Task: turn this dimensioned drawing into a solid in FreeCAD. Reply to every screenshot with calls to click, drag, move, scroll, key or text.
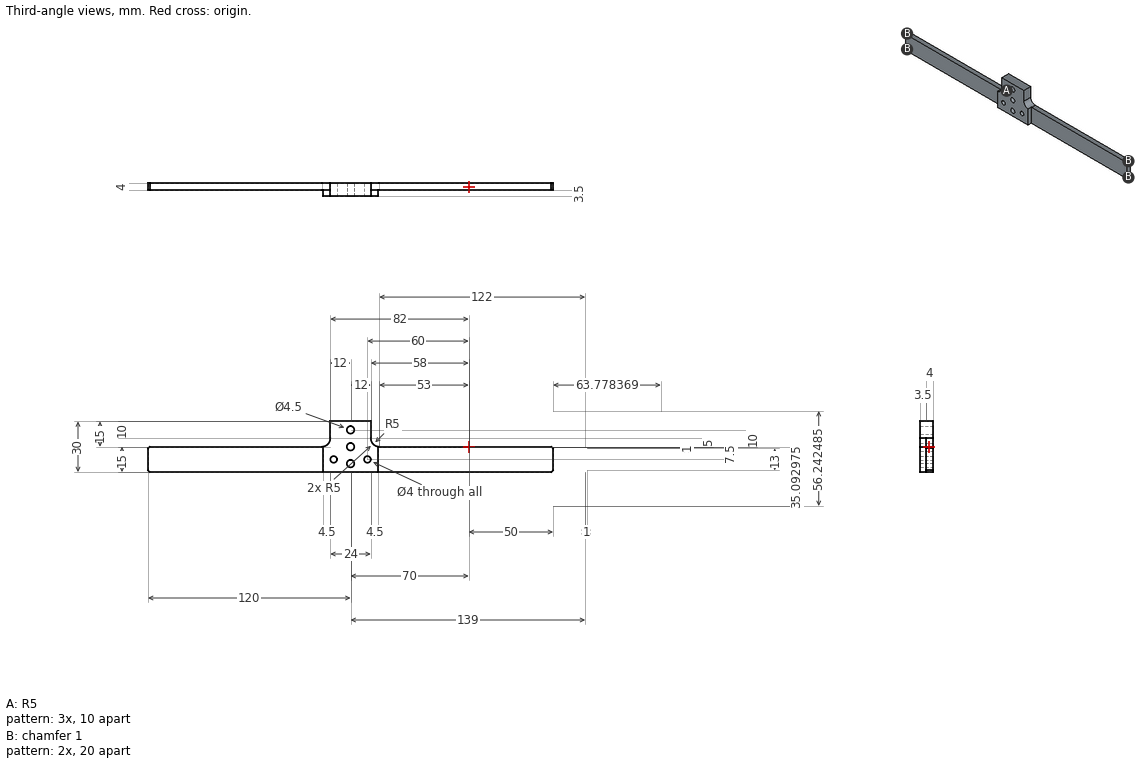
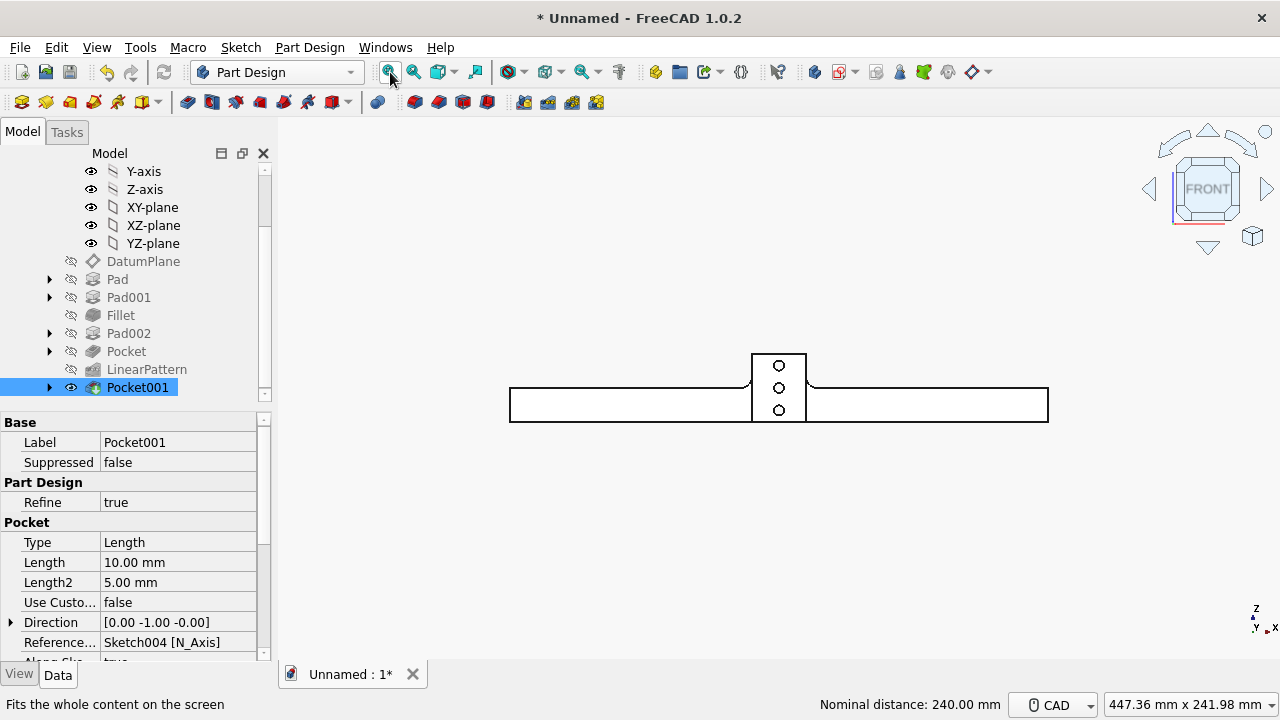
scroll(1048, 421, up, 8)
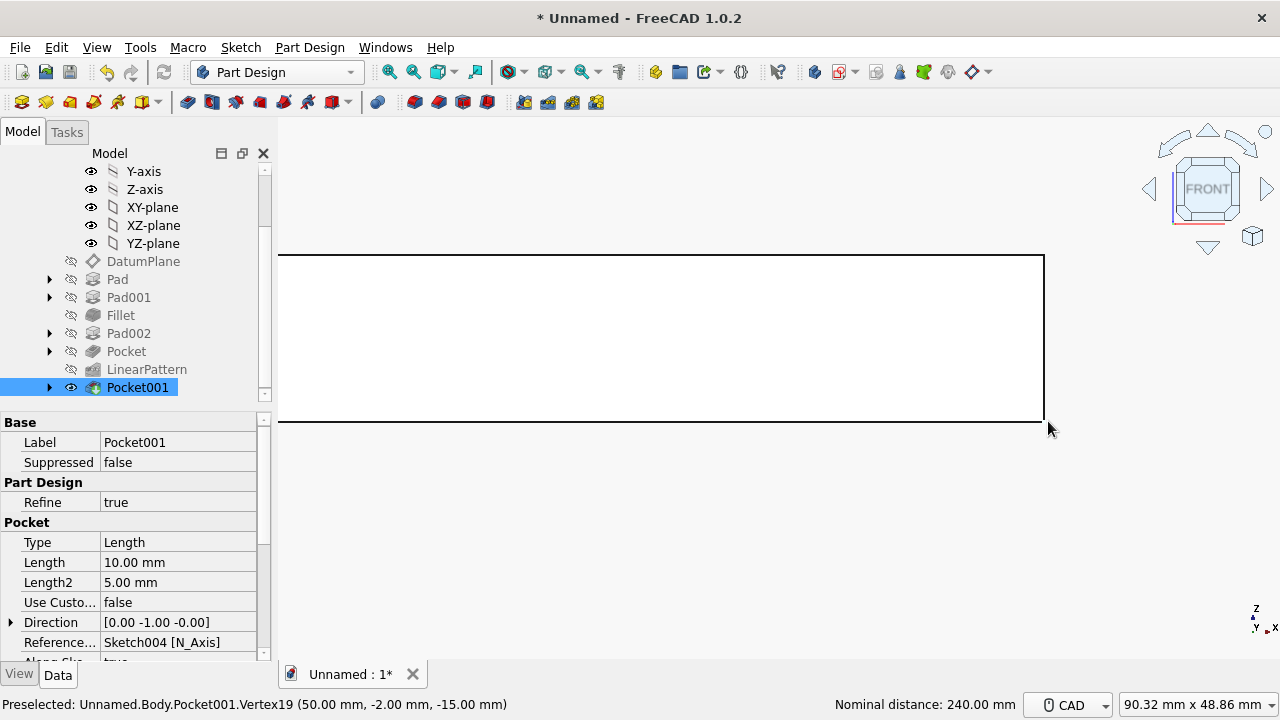
click(390, 72)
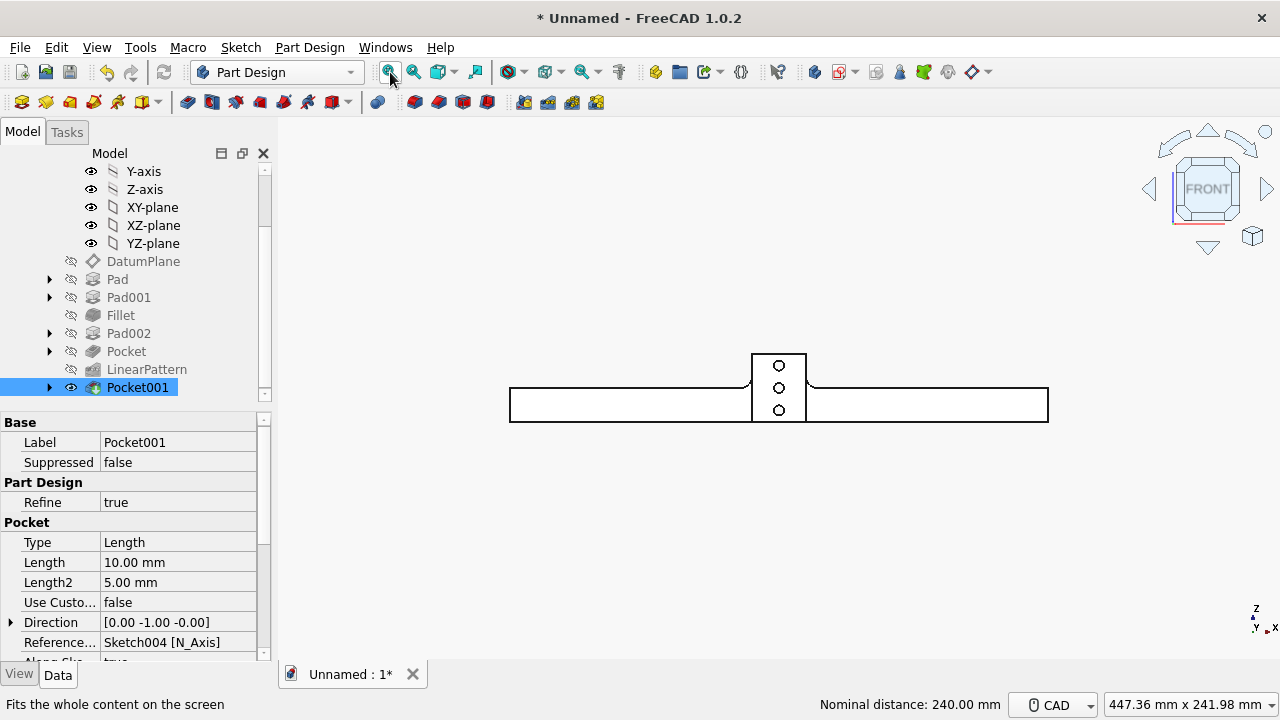
key(3)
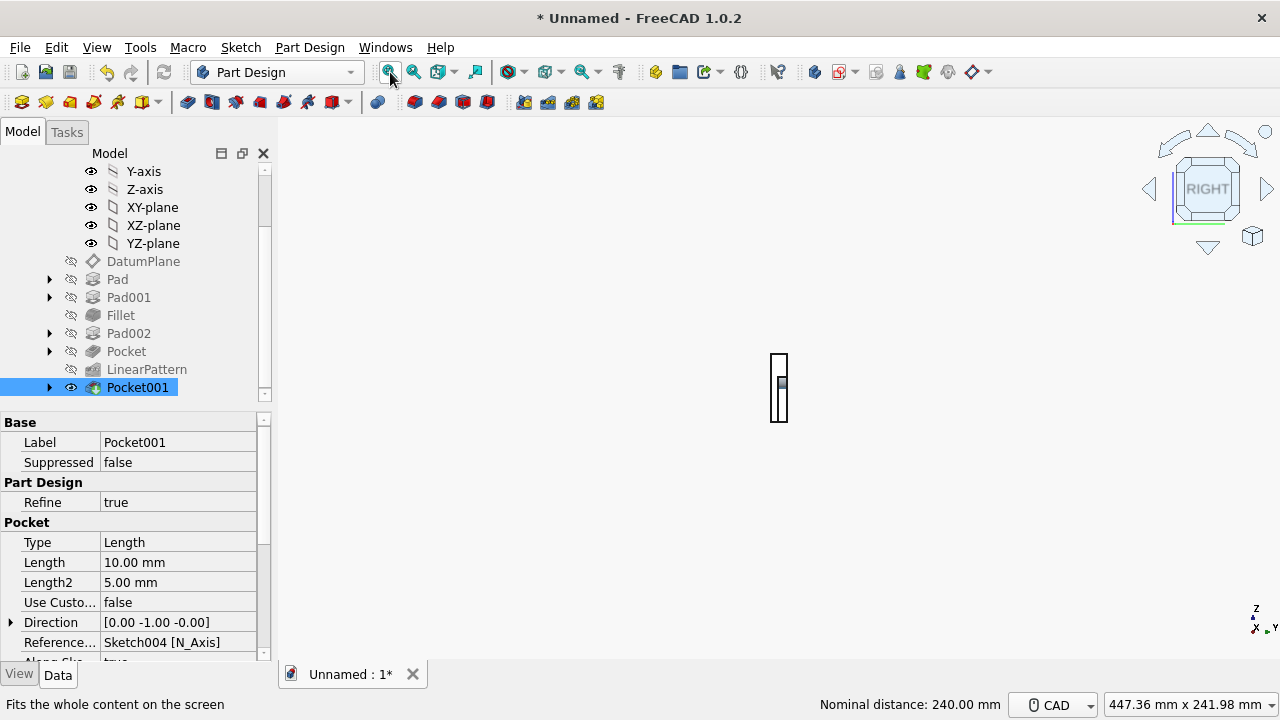
click(390, 72)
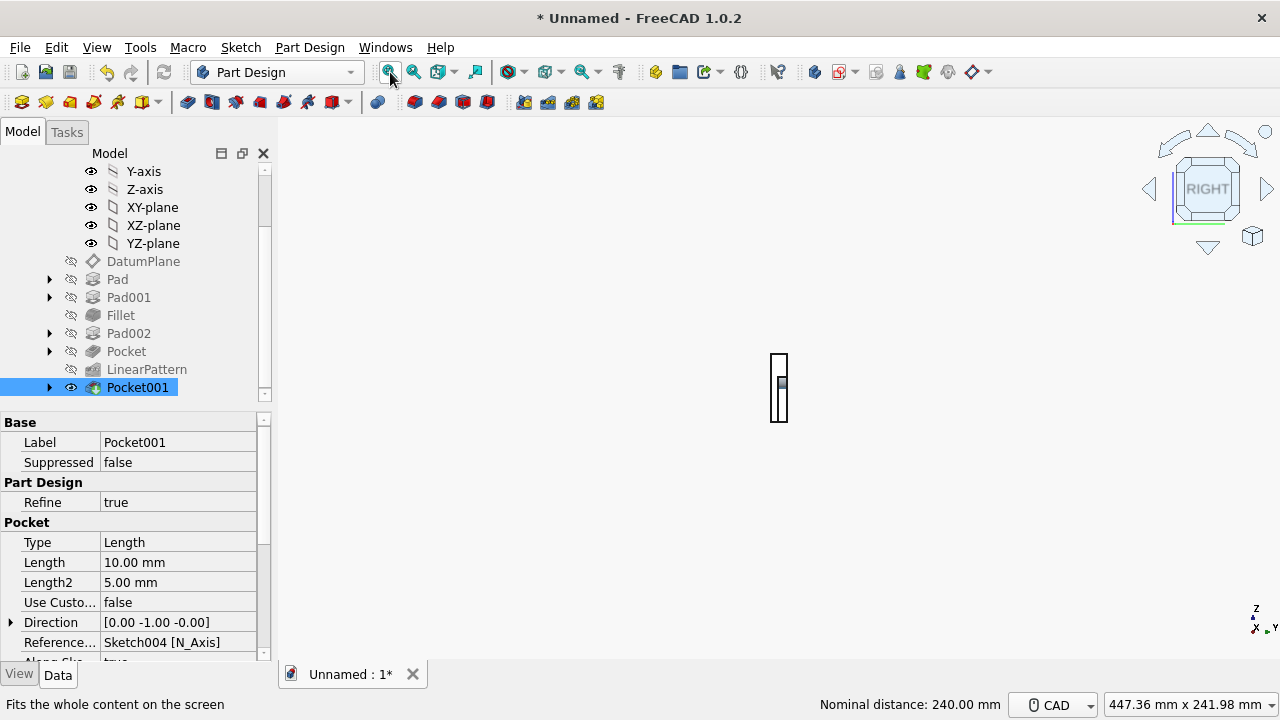
scroll(783, 421, up, 8)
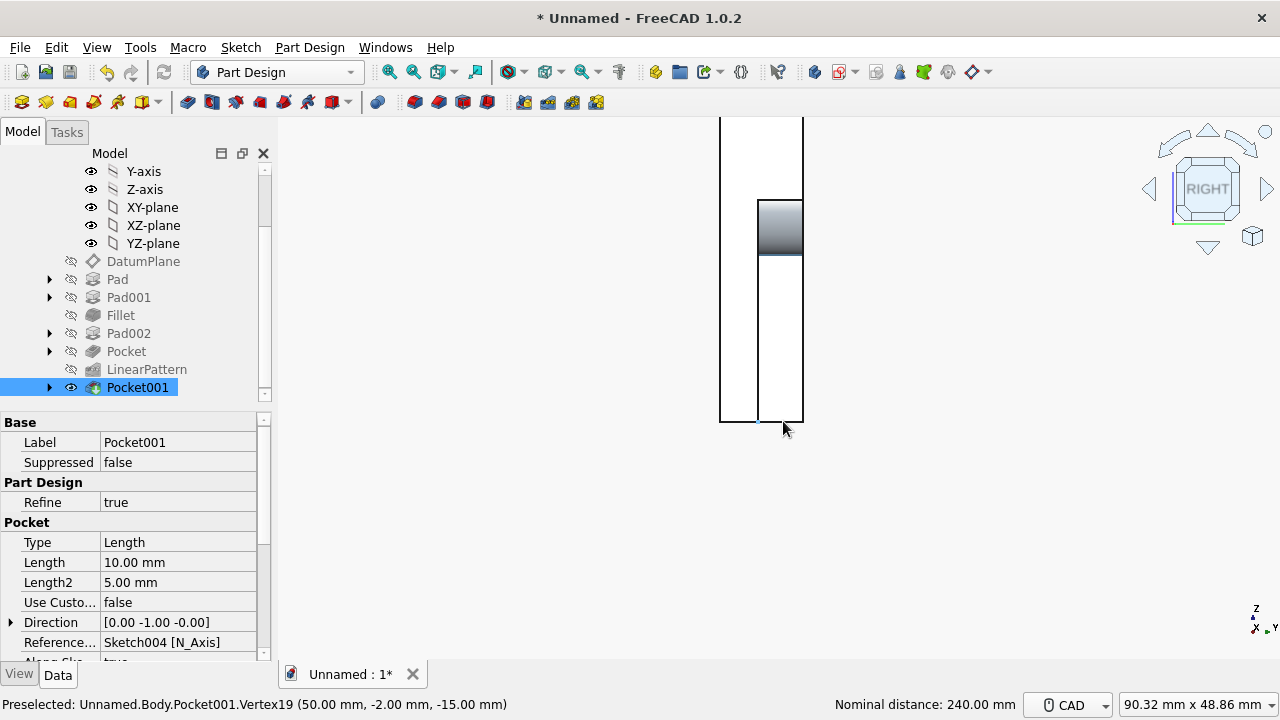
click(781, 421, ctrl)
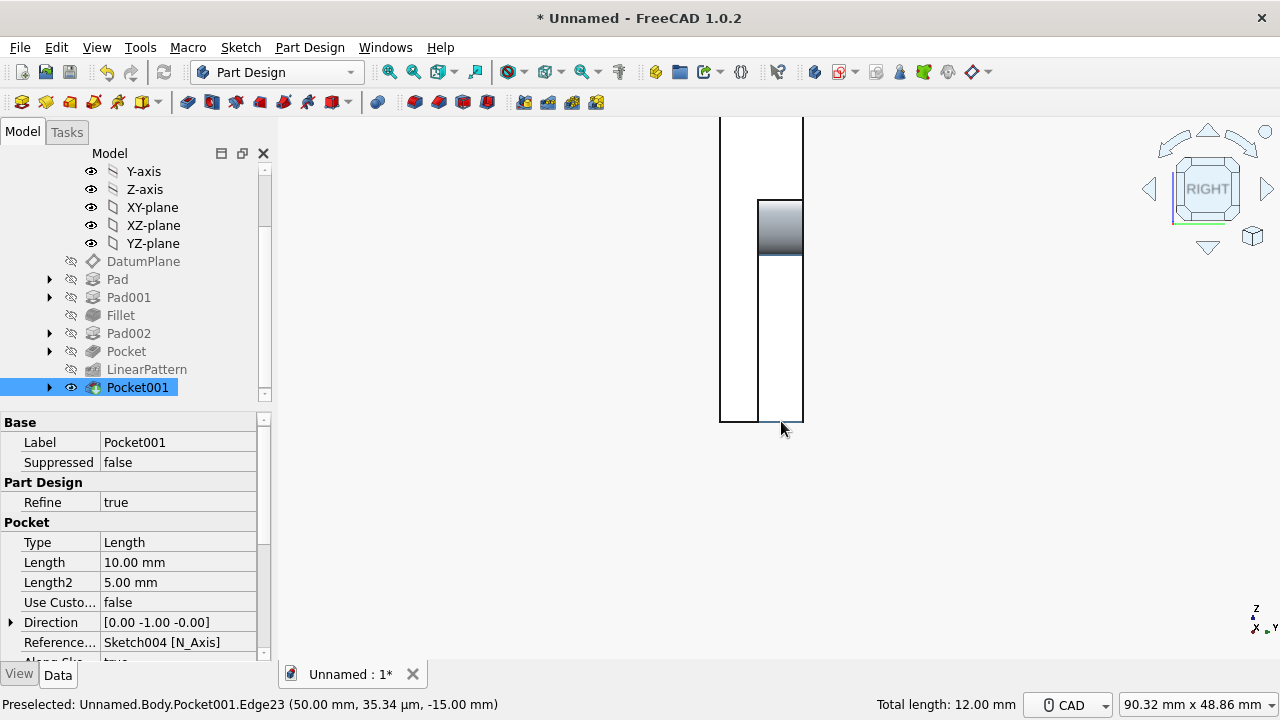
click(390, 72)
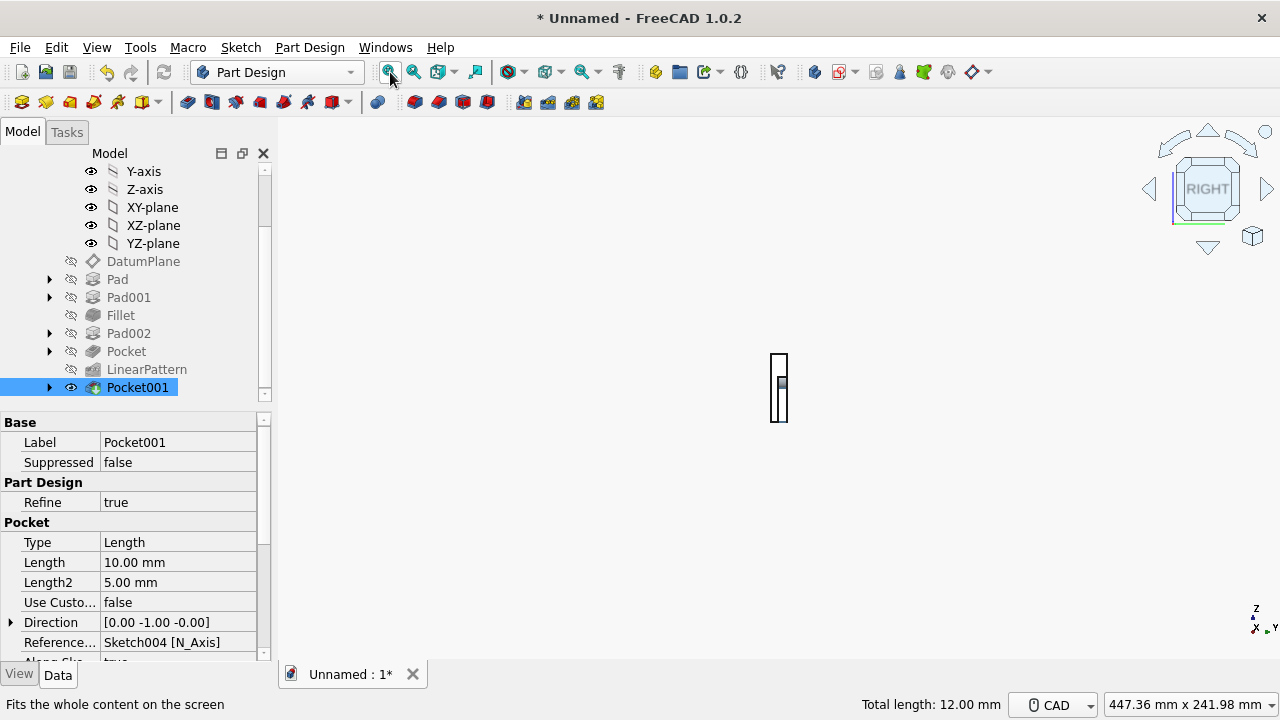
key(5)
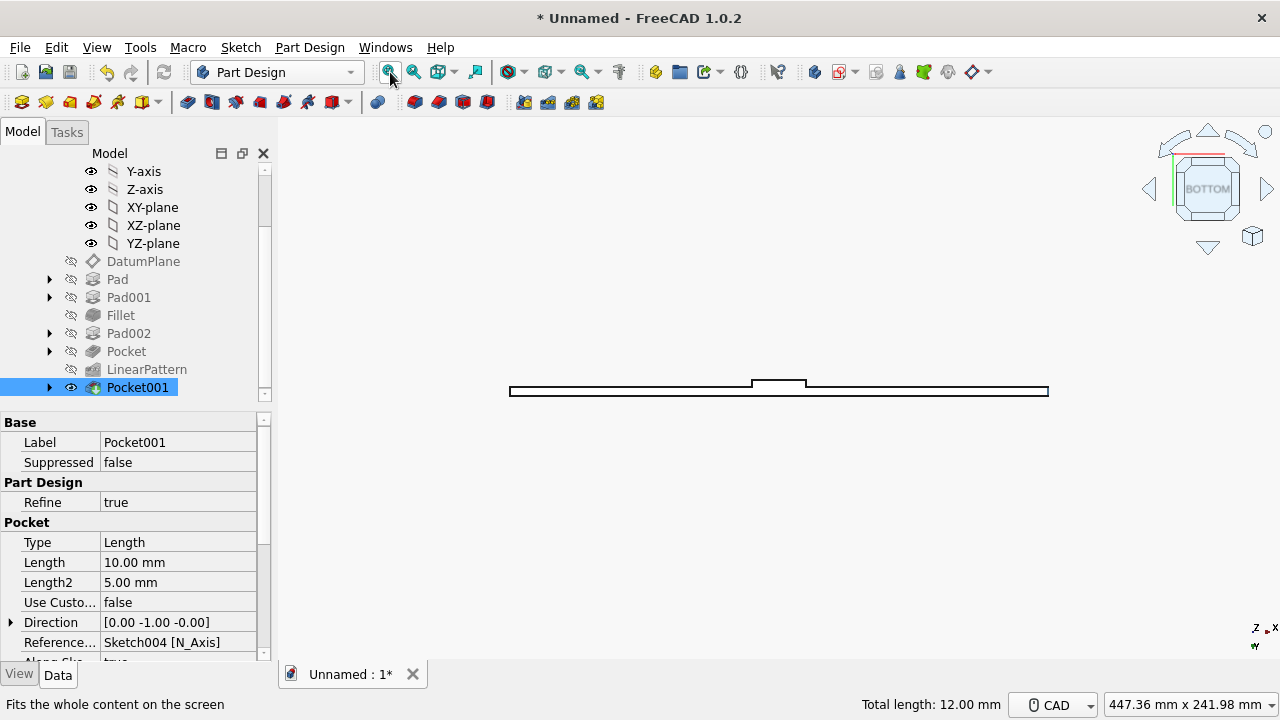
click(510, 393, ctrl)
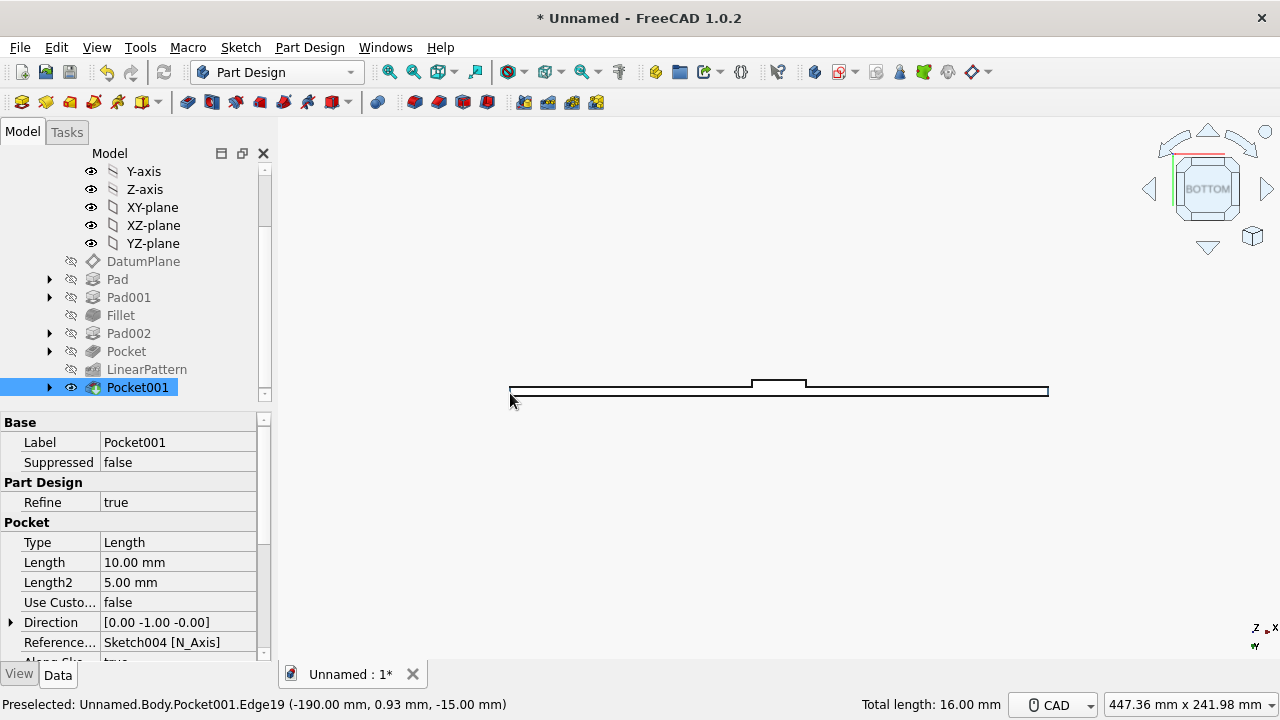
click(440, 102)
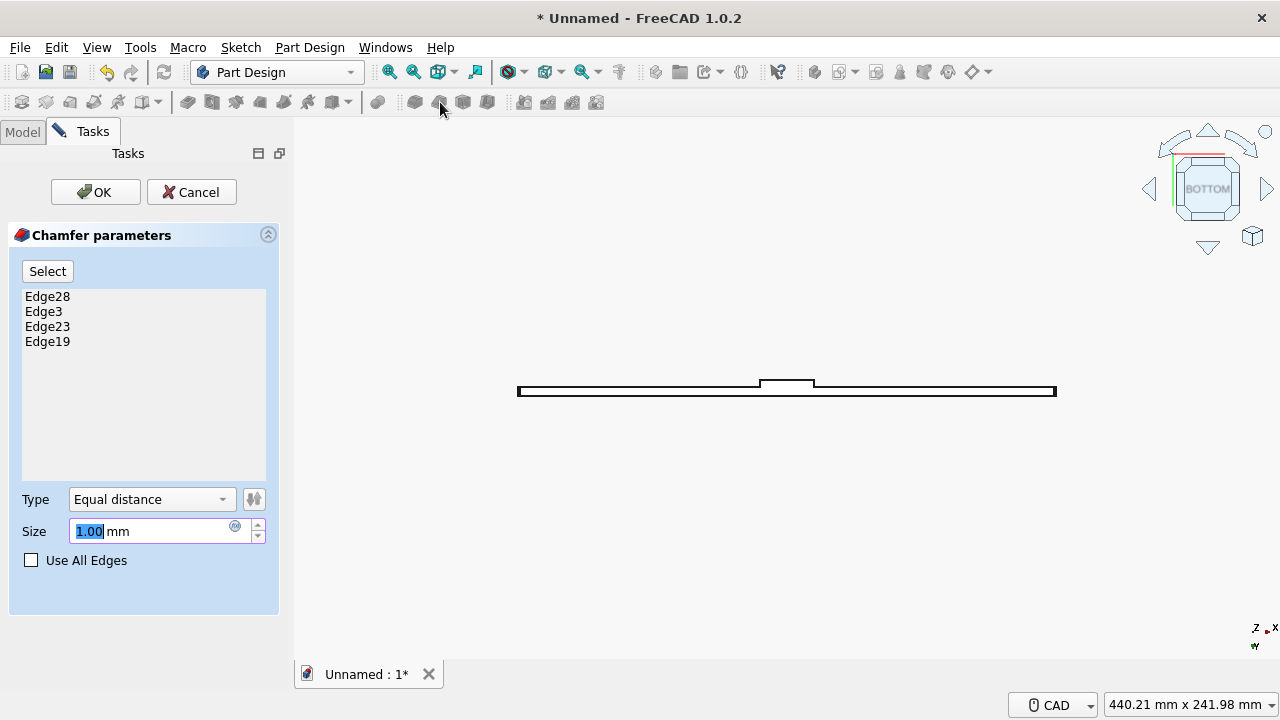
text(1)
key(Tab)